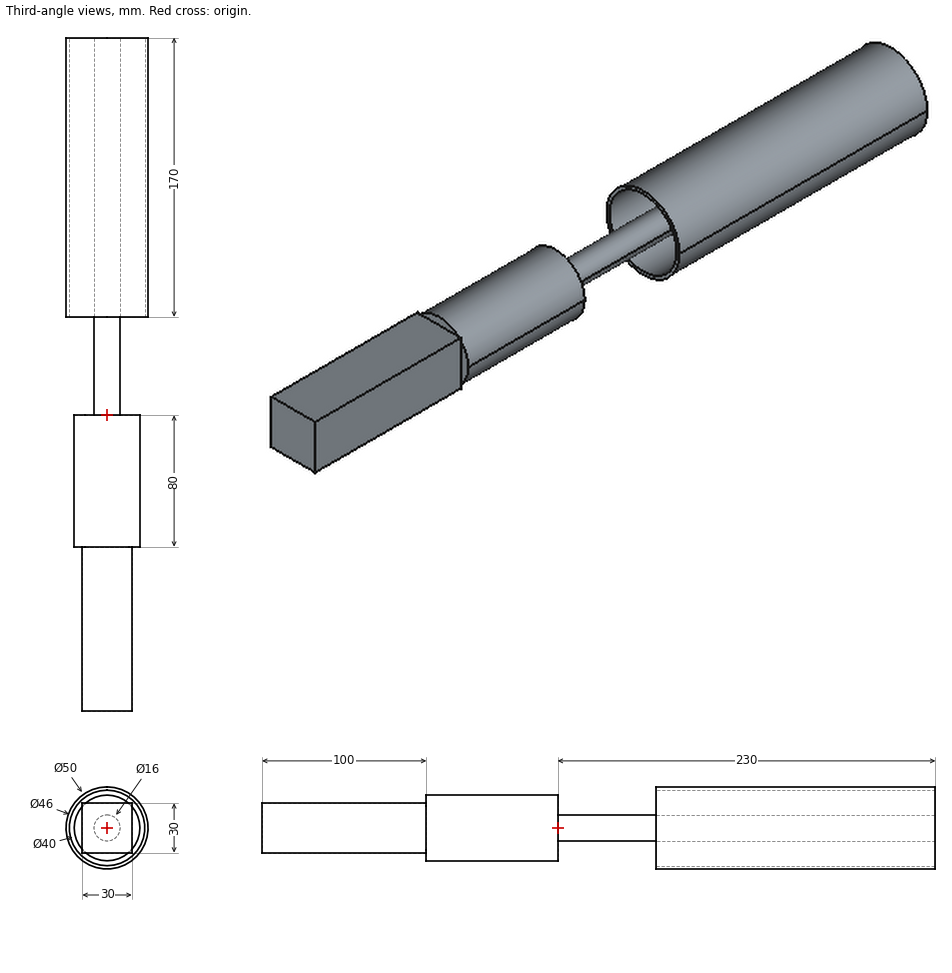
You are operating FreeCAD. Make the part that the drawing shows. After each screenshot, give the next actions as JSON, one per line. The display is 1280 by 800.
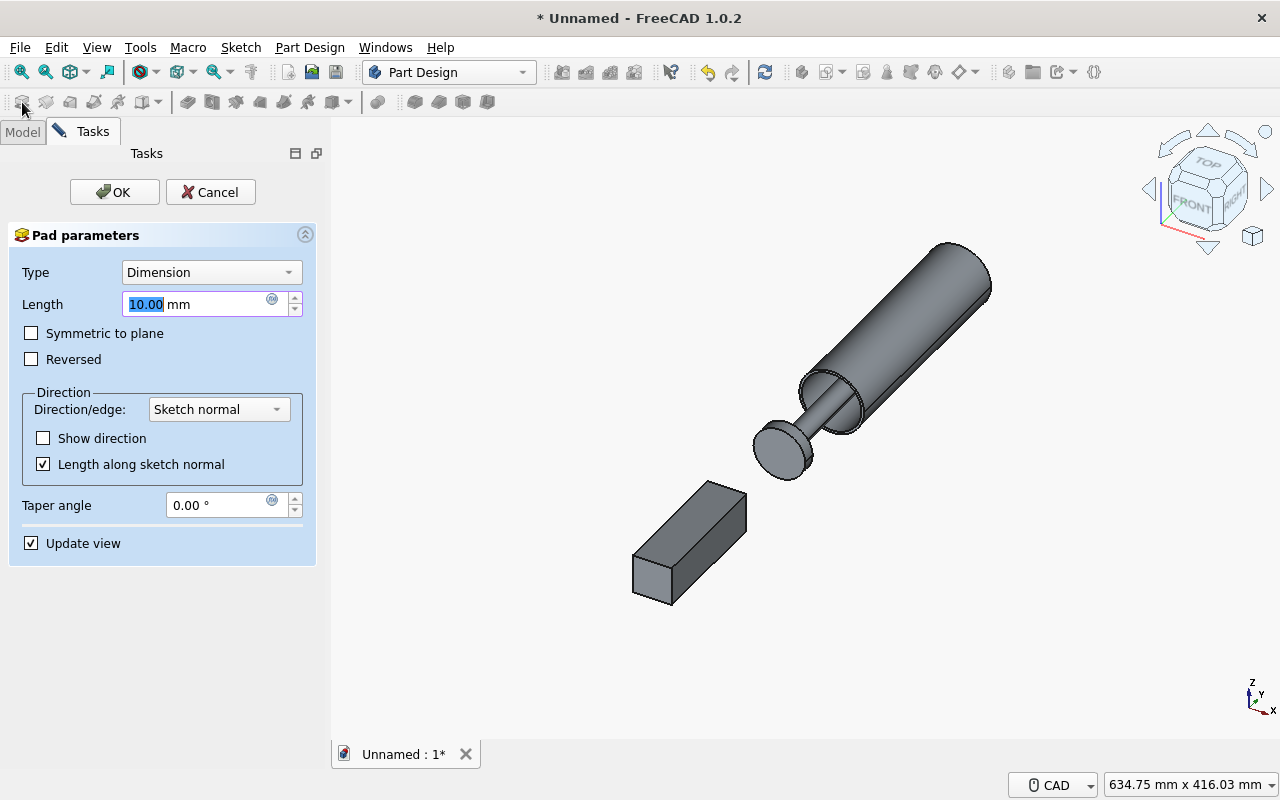
{"action": "type", "text": "80"}
{"action": "key", "text": "Tab"}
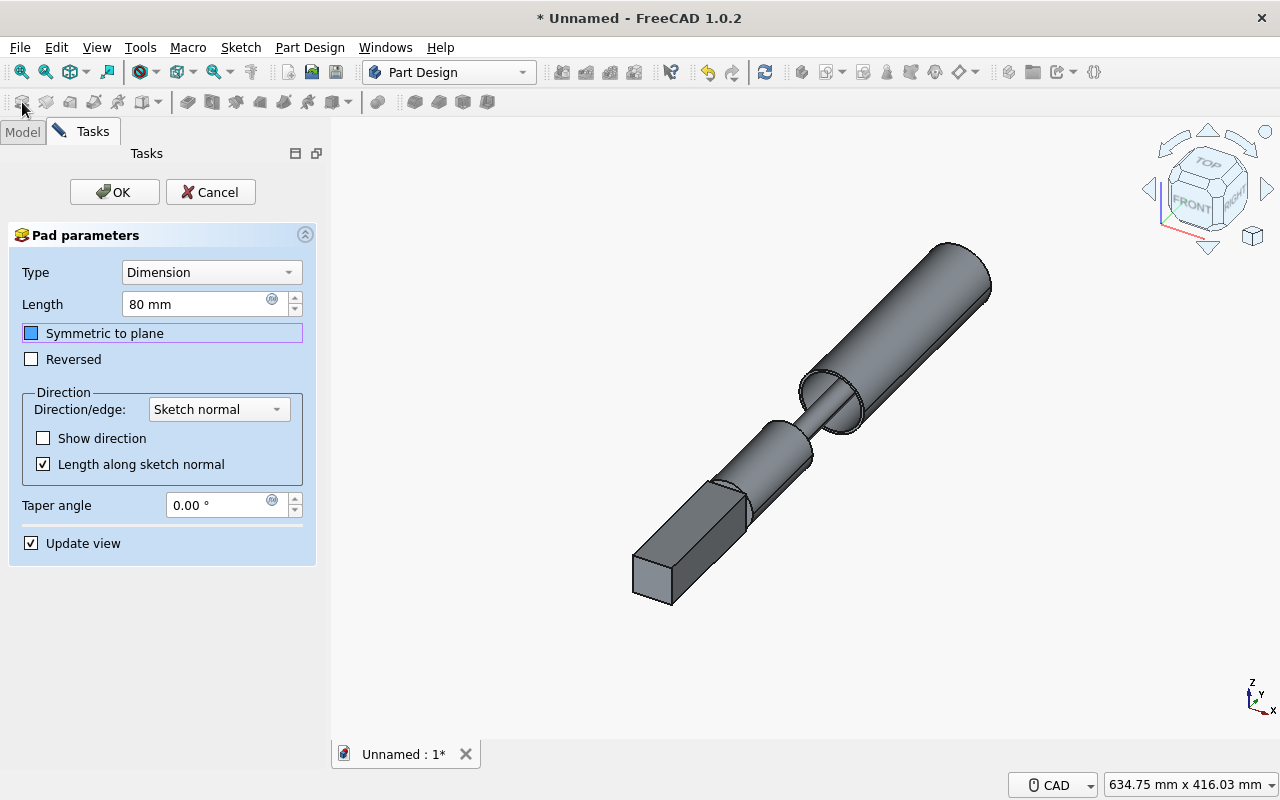
{"action": "left_click", "coordinate": [115, 192]}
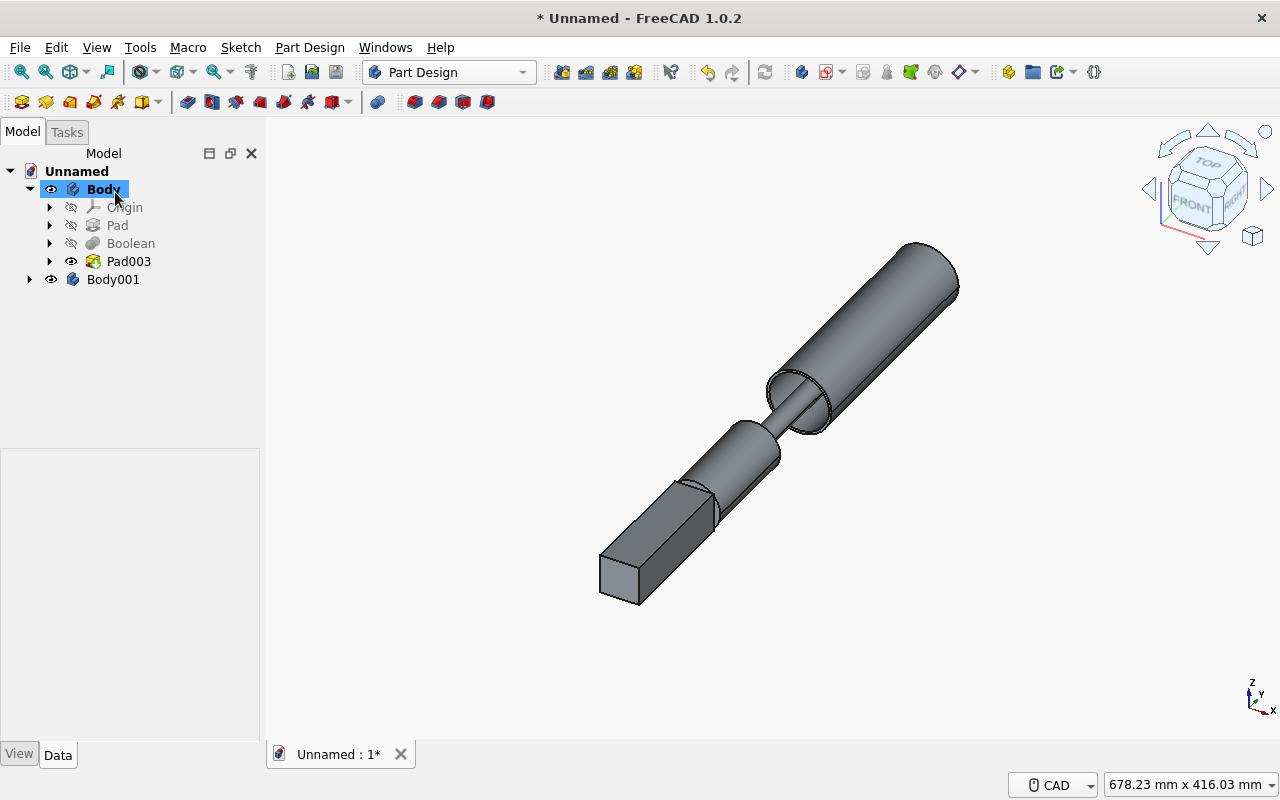
{"action": "key", "text": "0"}